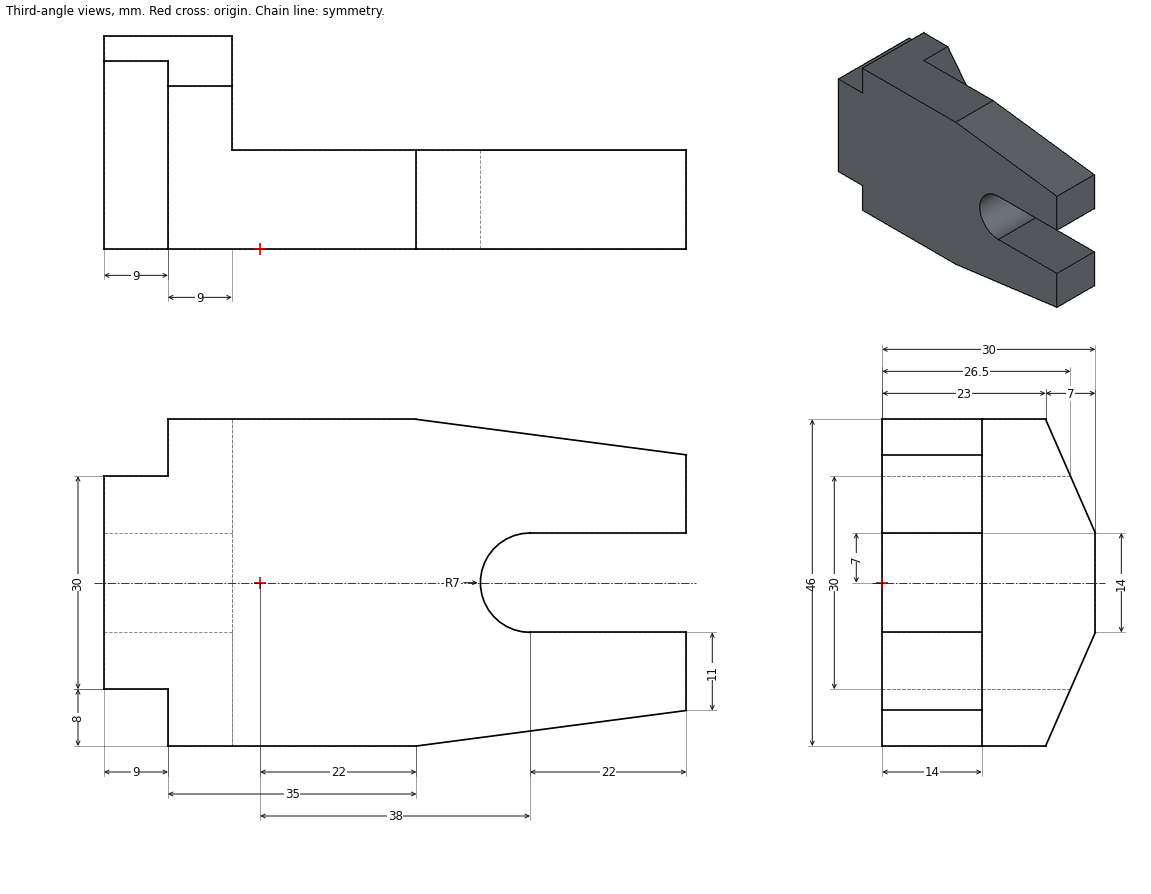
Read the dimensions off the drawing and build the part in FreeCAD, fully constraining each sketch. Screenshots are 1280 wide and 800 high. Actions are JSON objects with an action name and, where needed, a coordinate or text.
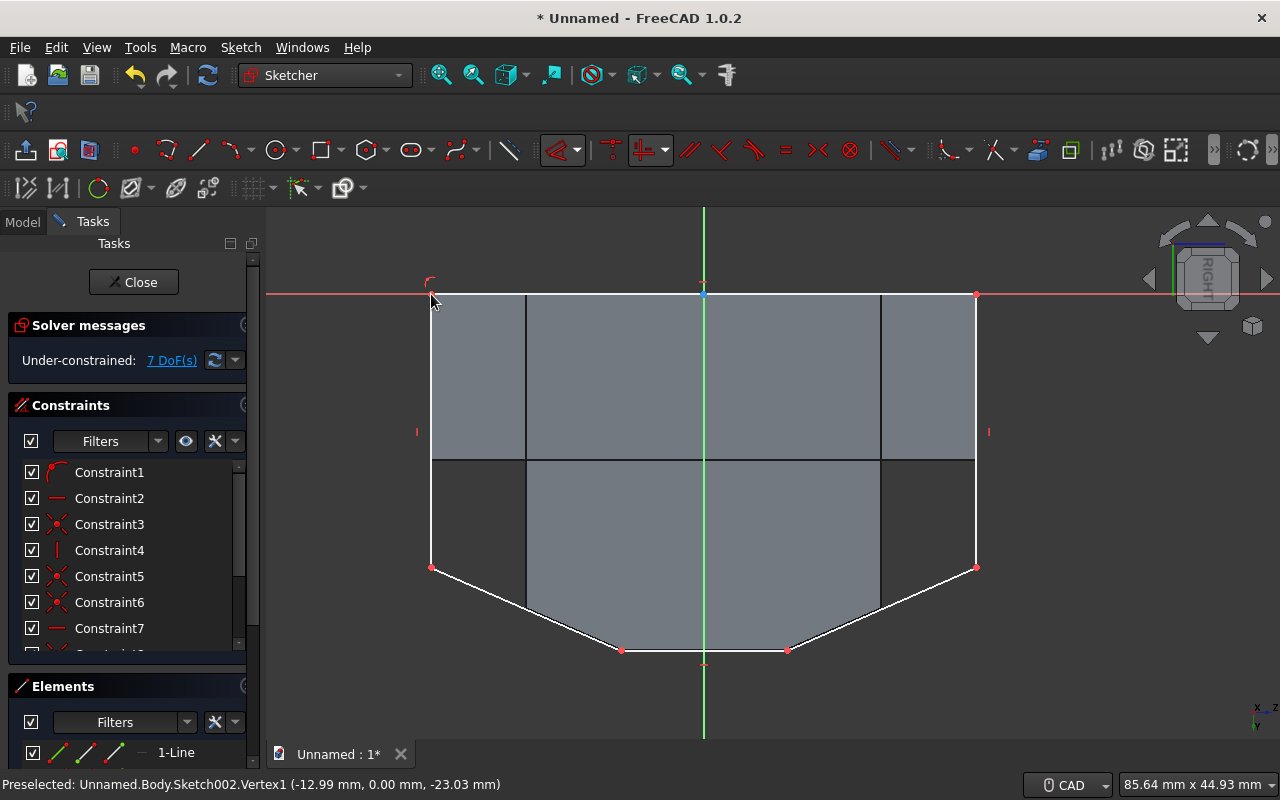
{"action": "left_click", "coordinate": [976, 568]}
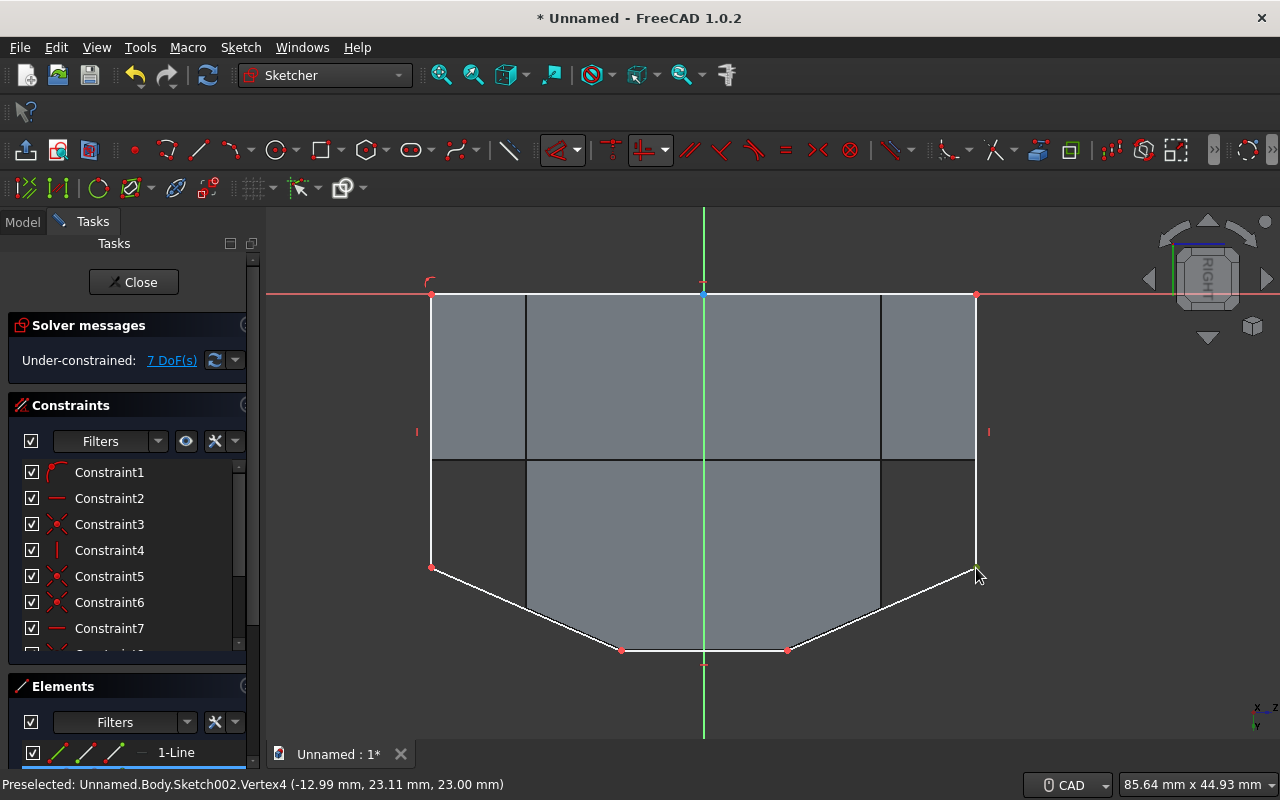
{"action": "left_click", "coordinate": [431, 568]}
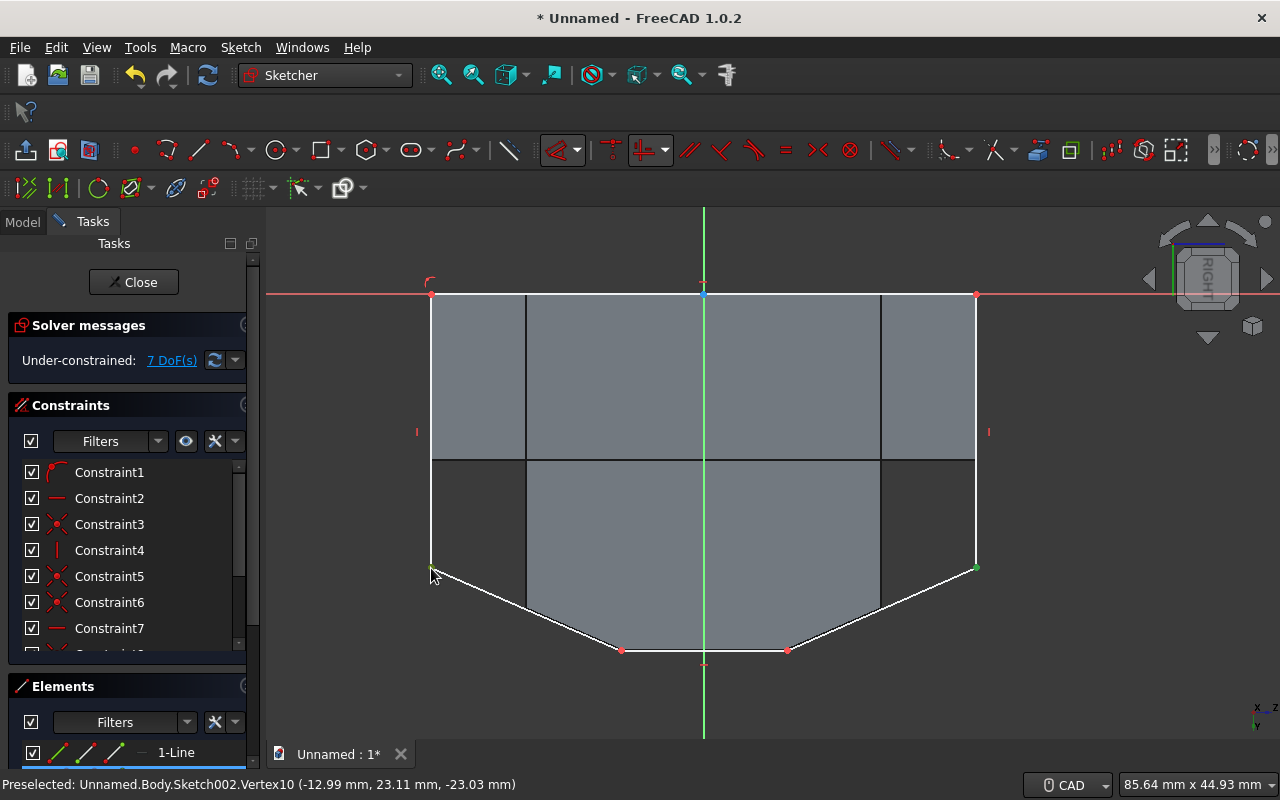
{"action": "left_click", "coordinate": [704, 609]}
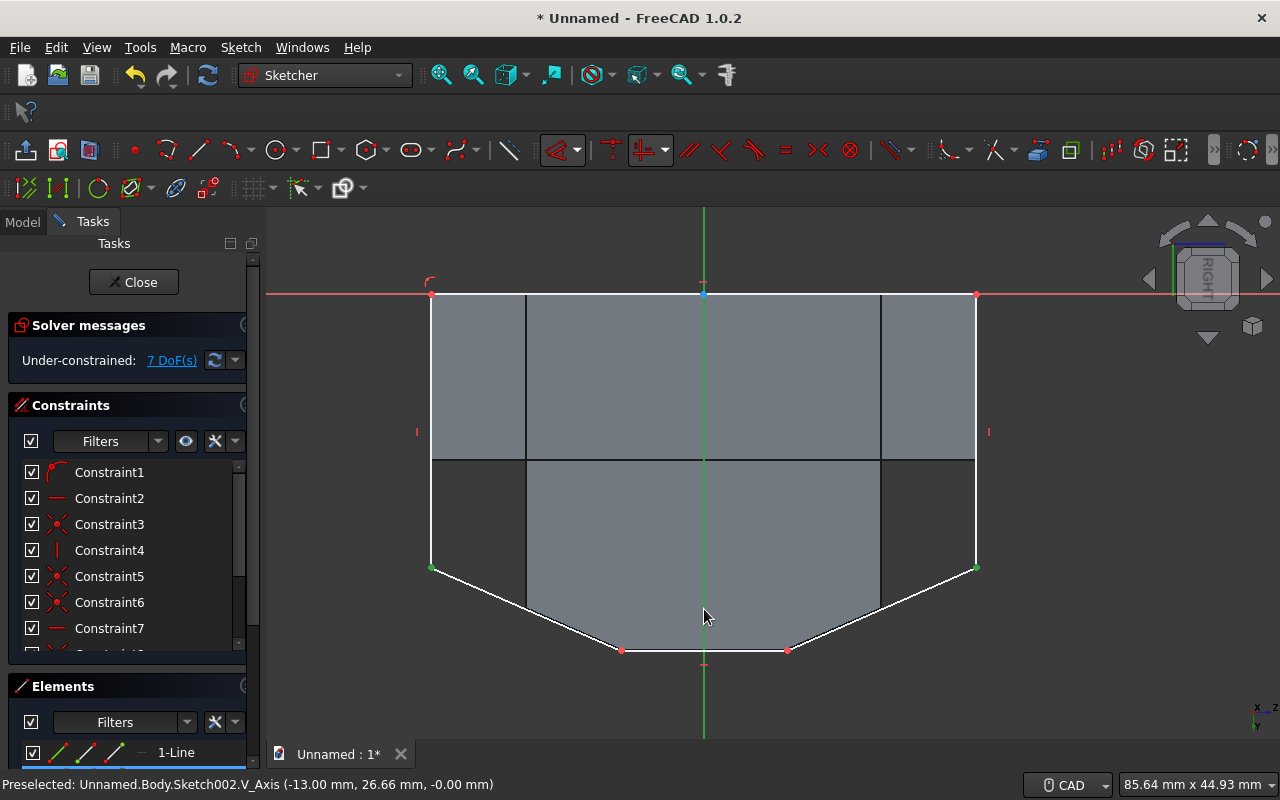
{"action": "left_click", "coordinate": [818, 150]}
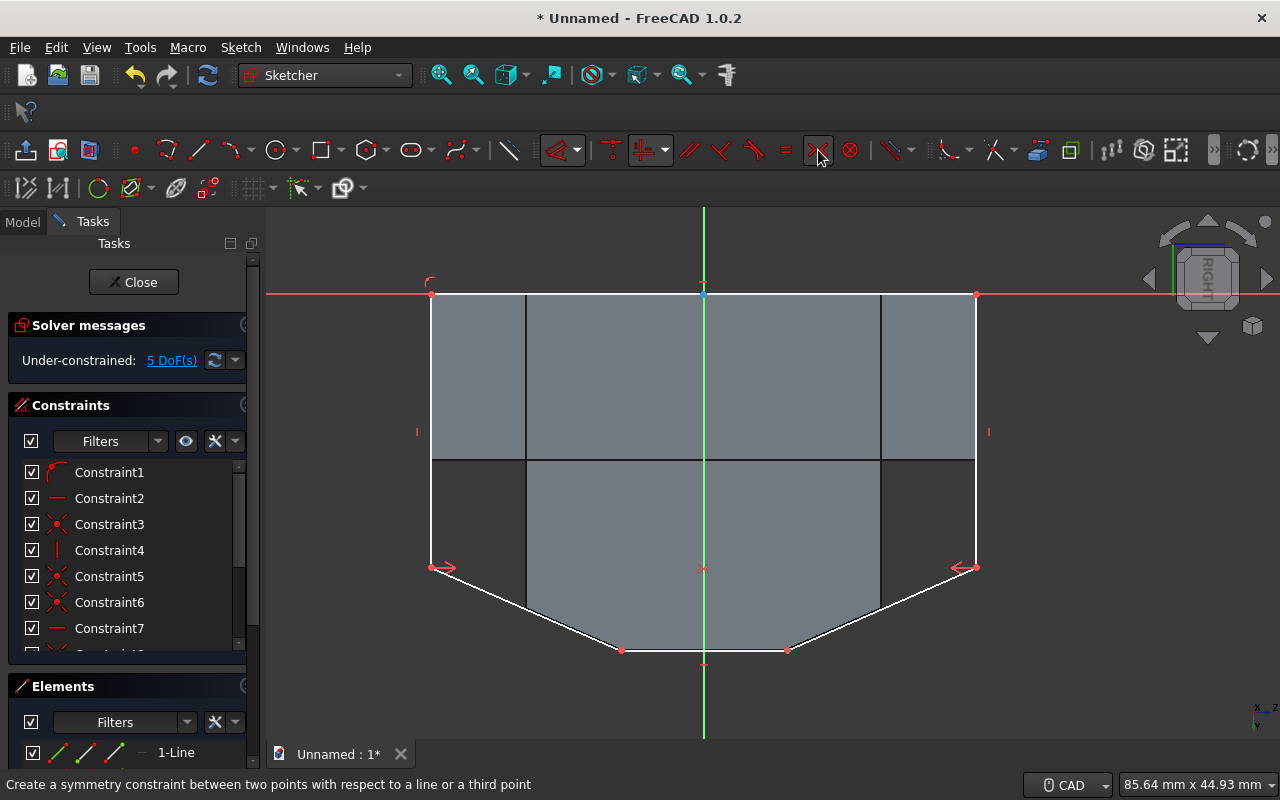
{"action": "key", "text": "d"}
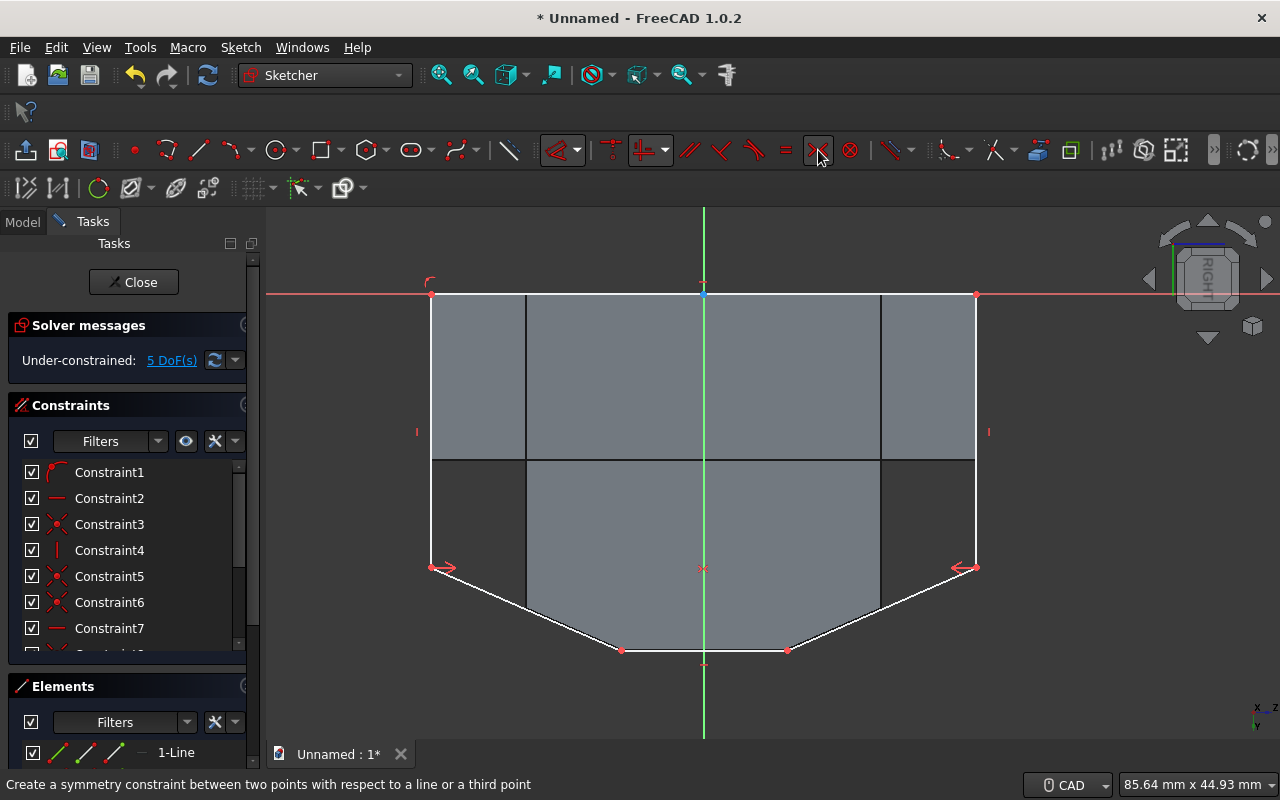
{"action": "left_click", "coordinate": [595, 294]}
{"action": "left_click", "coordinate": [578, 260]}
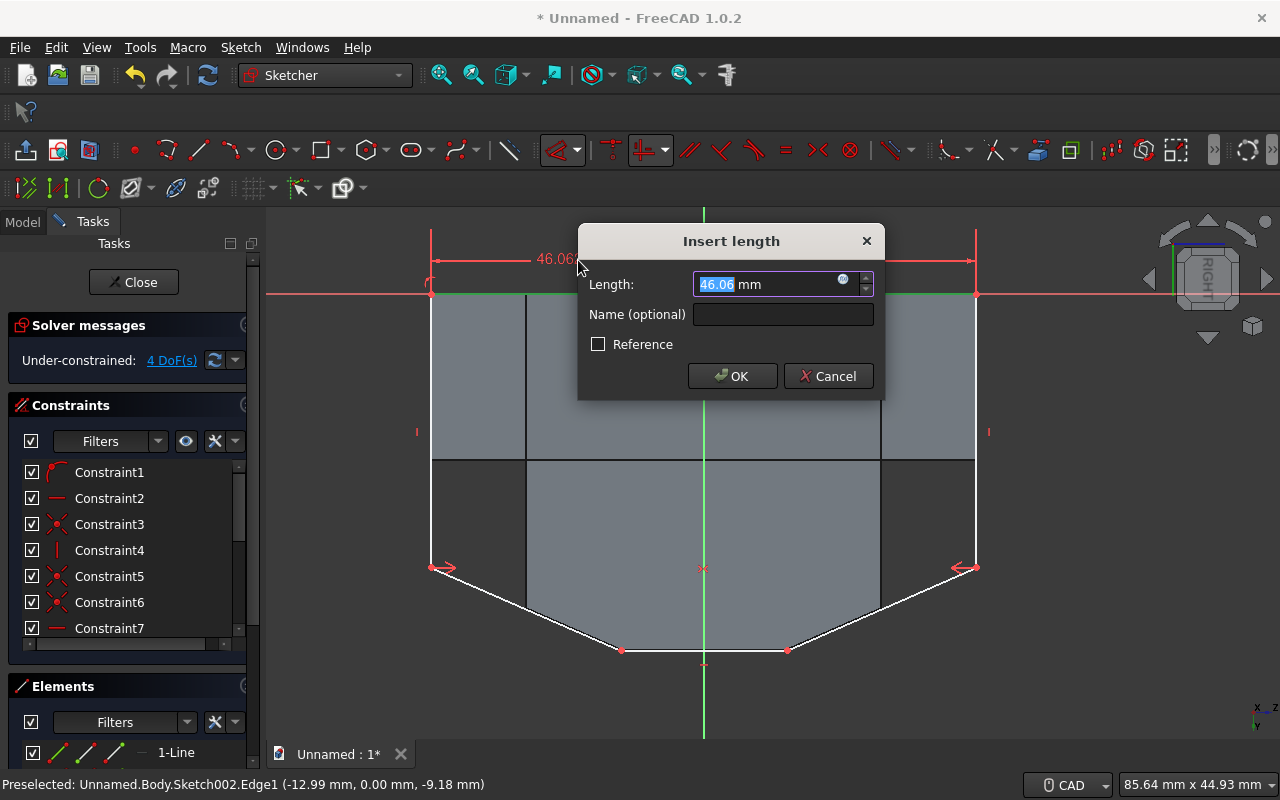
{"action": "type", "text": "46"}
{"action": "key", "text": "Return"}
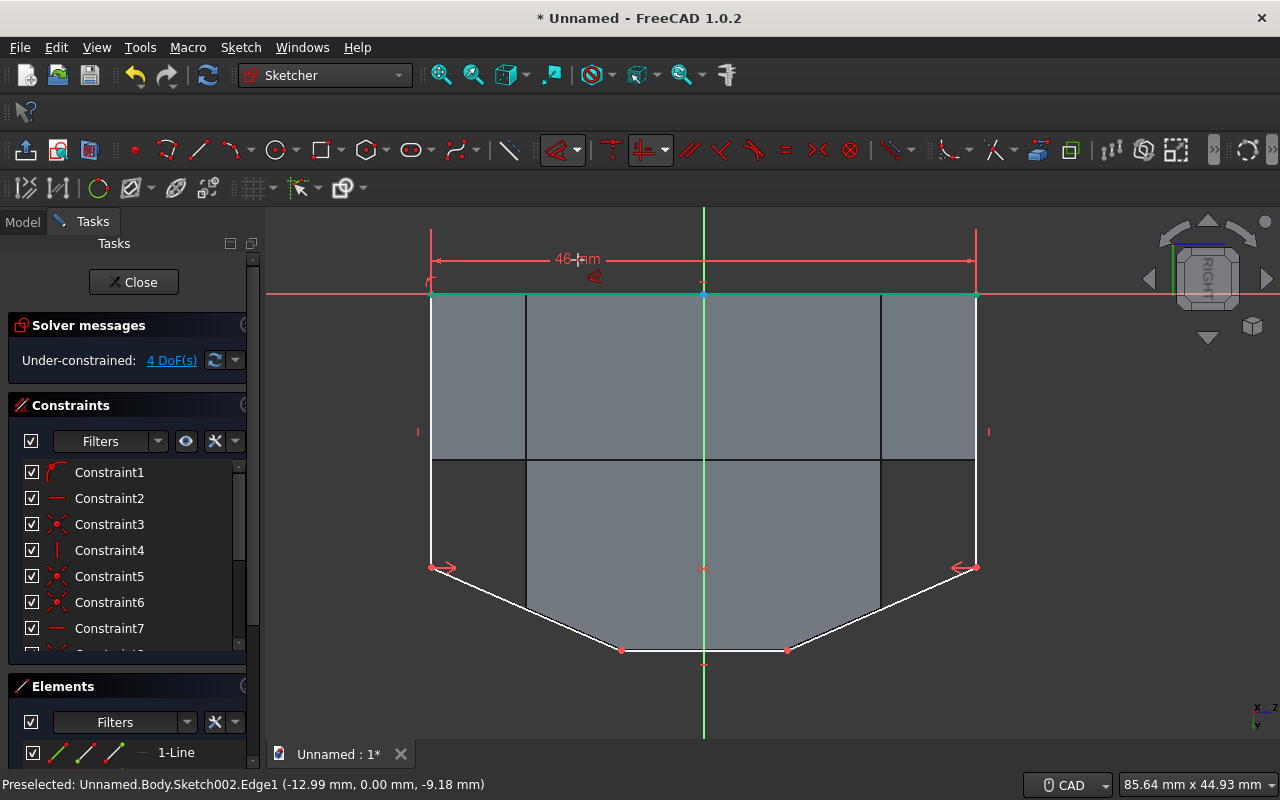
{"action": "left_click", "coordinate": [976, 376]}
{"action": "left_click", "coordinate": [1010, 431]}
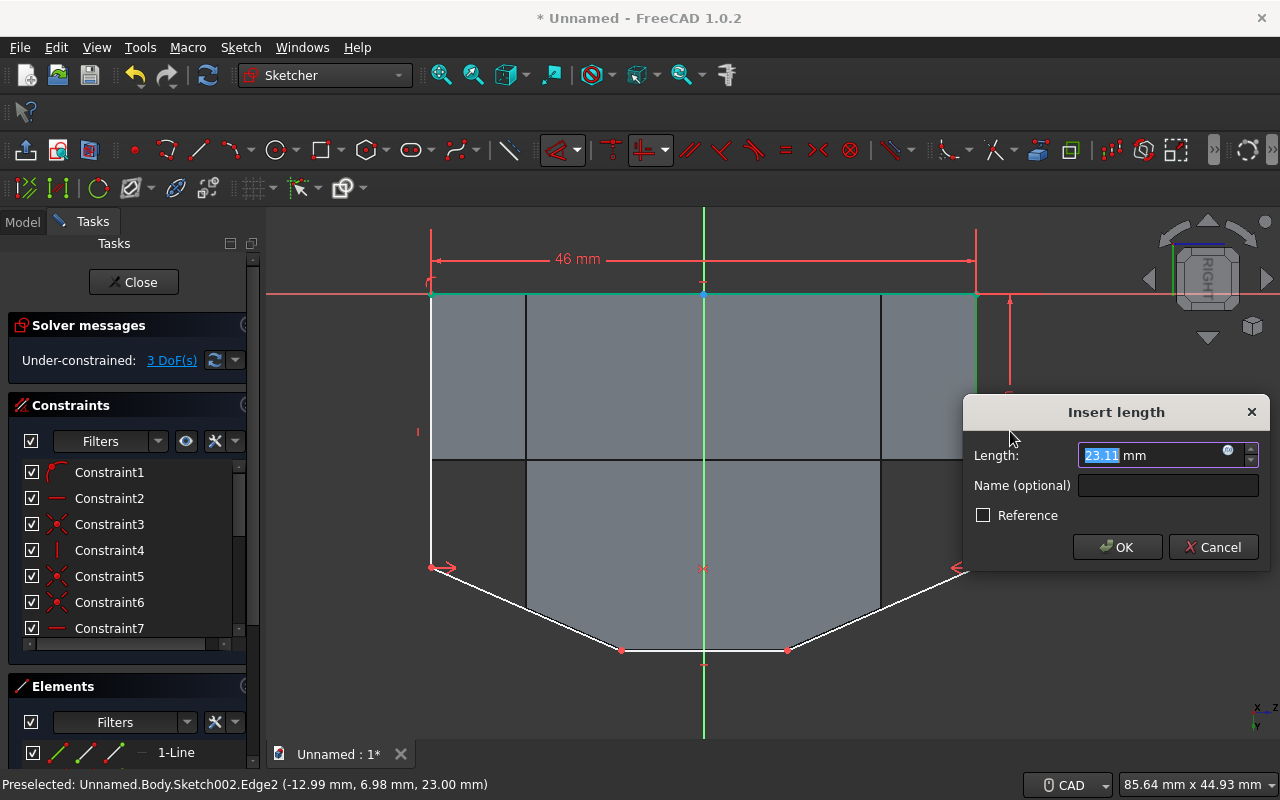
{"action": "type", "text": "23"}
{"action": "key", "text": "Return"}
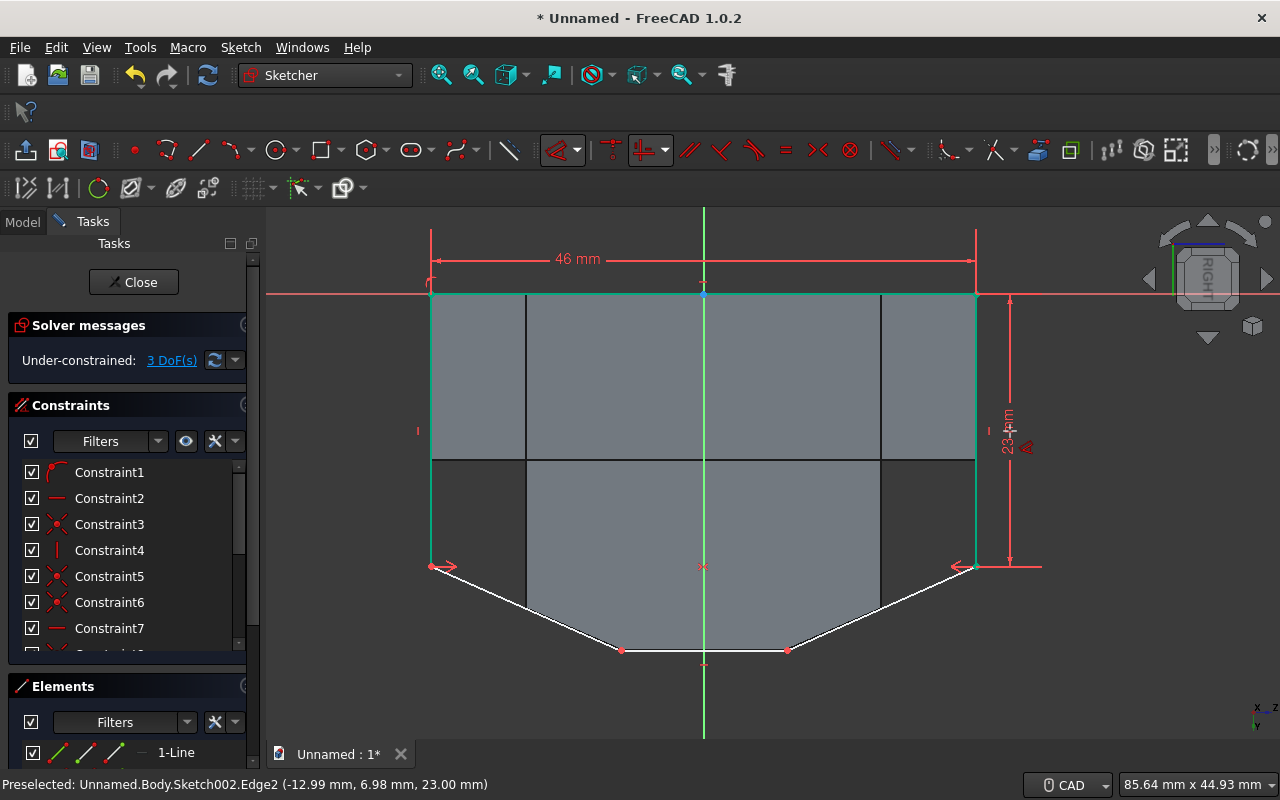
{"action": "left_click", "coordinate": [737, 651]}
{"action": "left_click", "coordinate": [666, 685]}